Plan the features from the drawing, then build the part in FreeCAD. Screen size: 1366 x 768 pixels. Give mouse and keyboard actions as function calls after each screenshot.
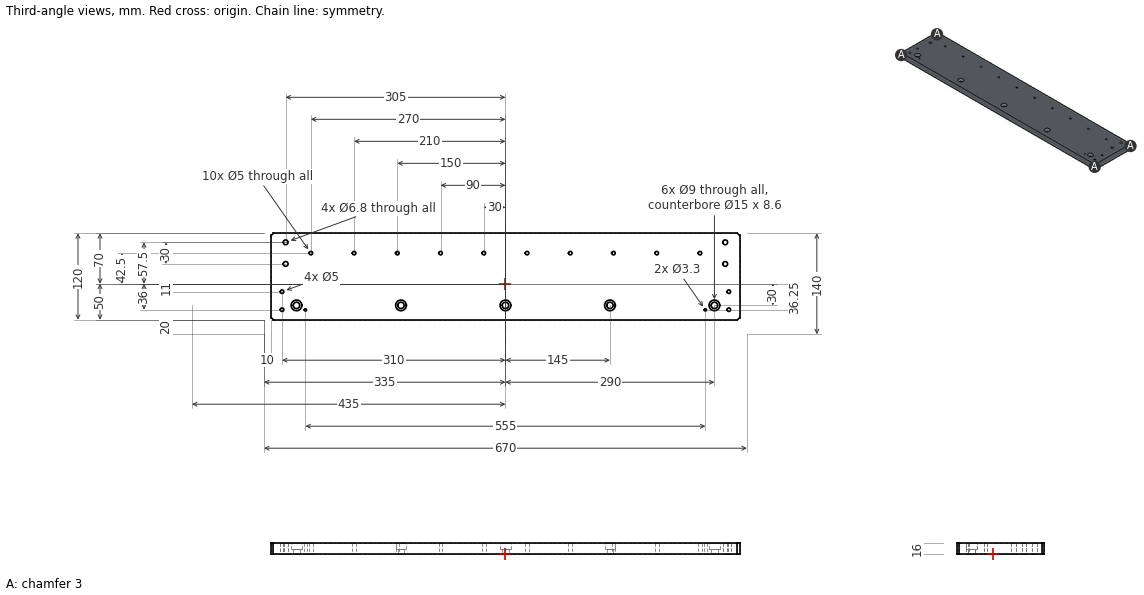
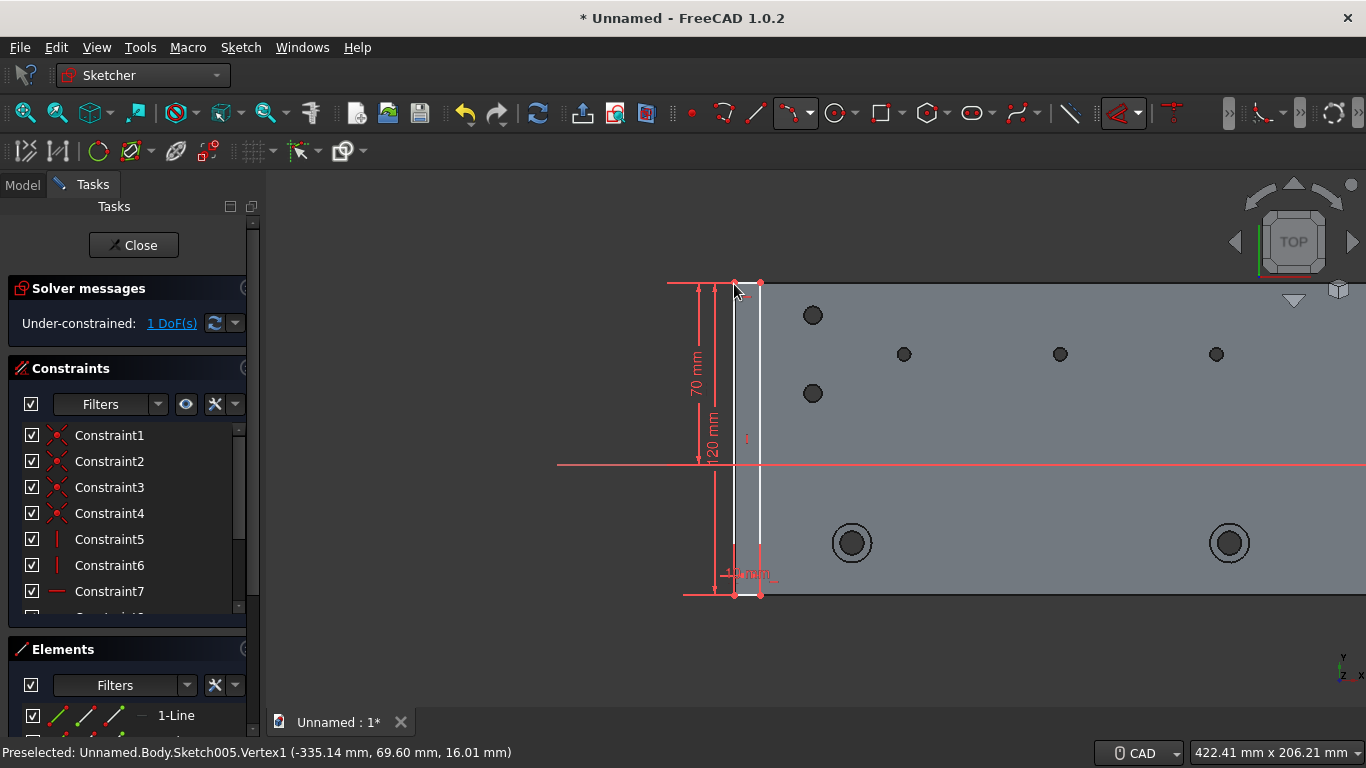
click(734, 283)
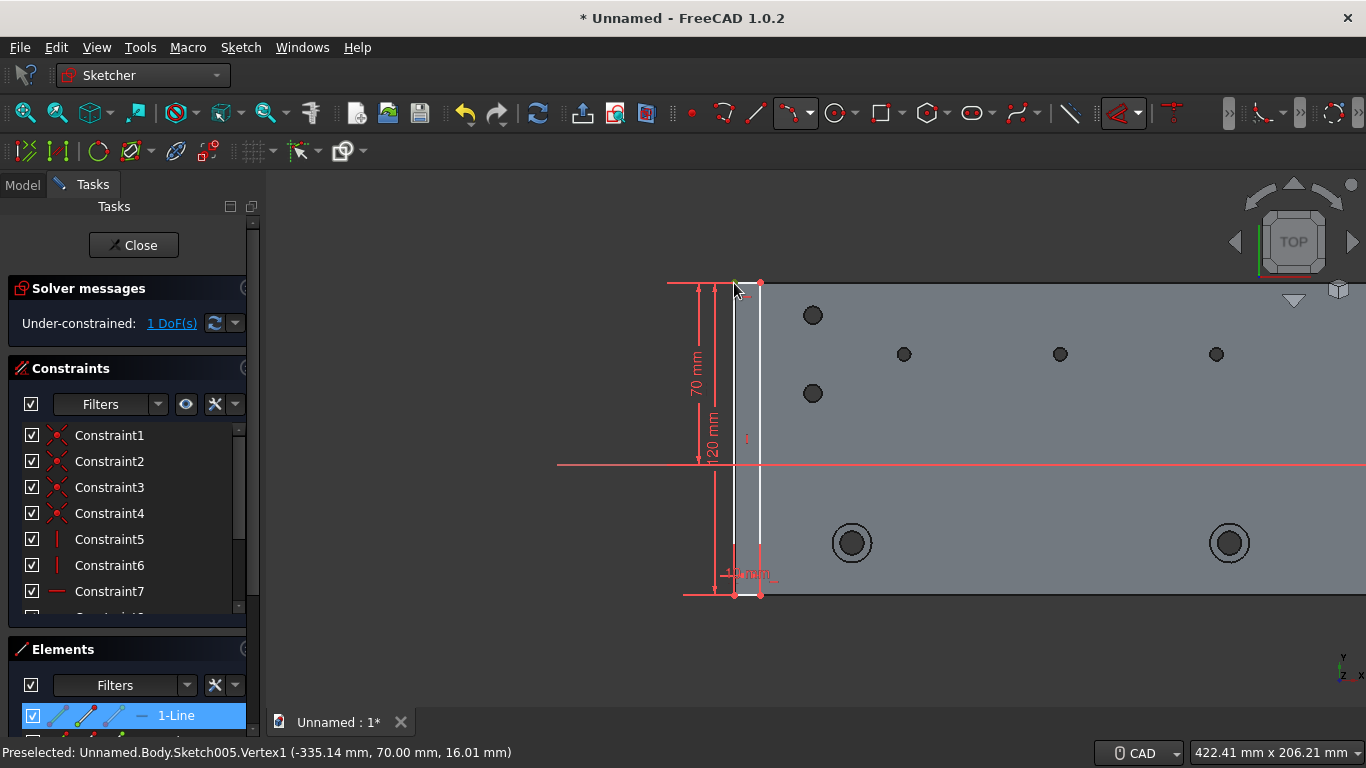
click(1140, 114)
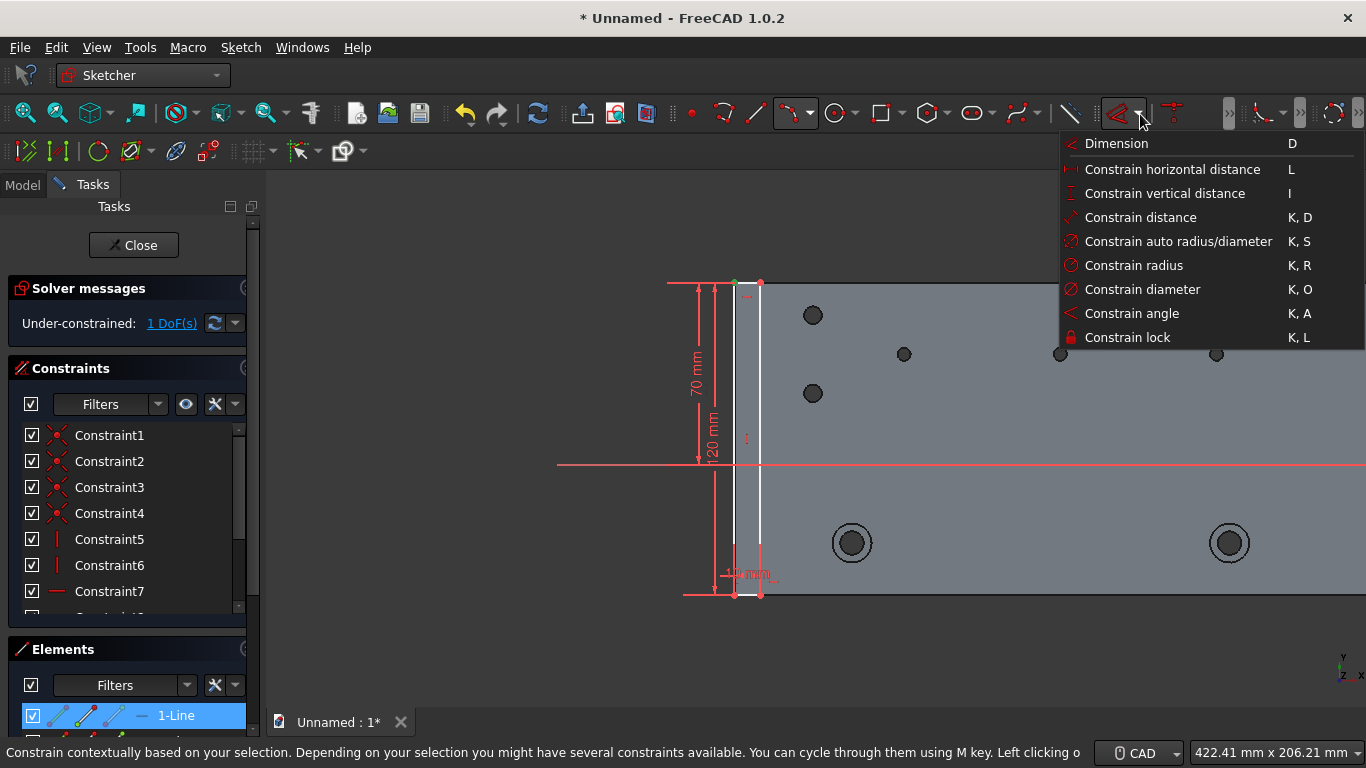
click(1212, 169)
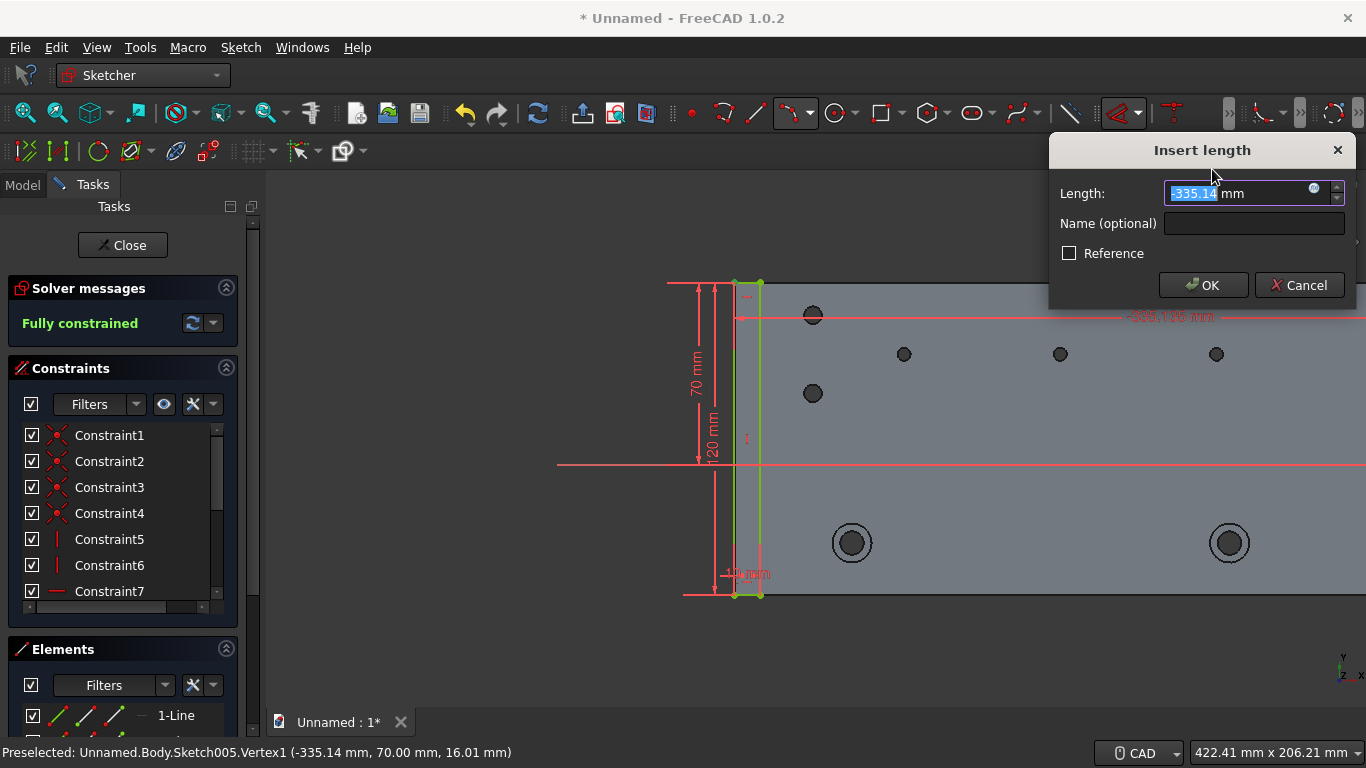
text(-335)
key(Return)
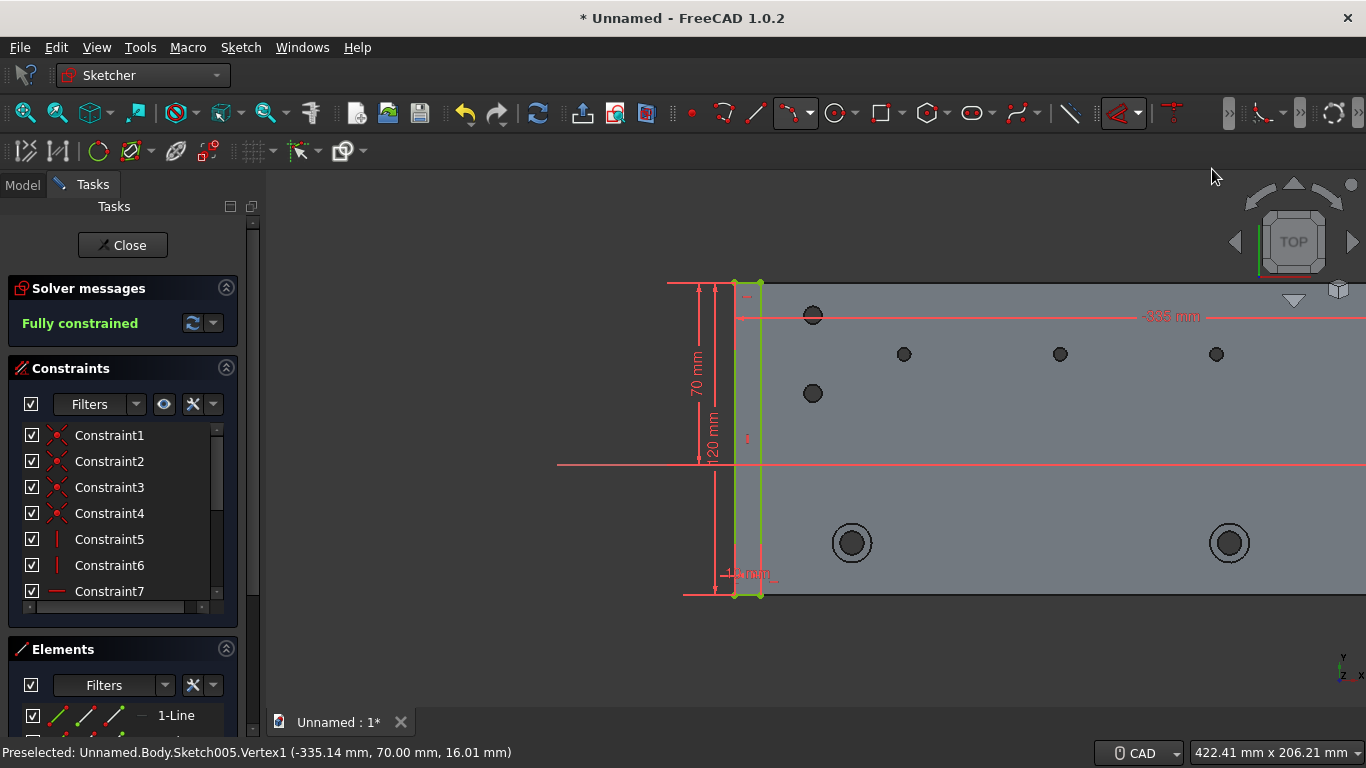
click(123, 245)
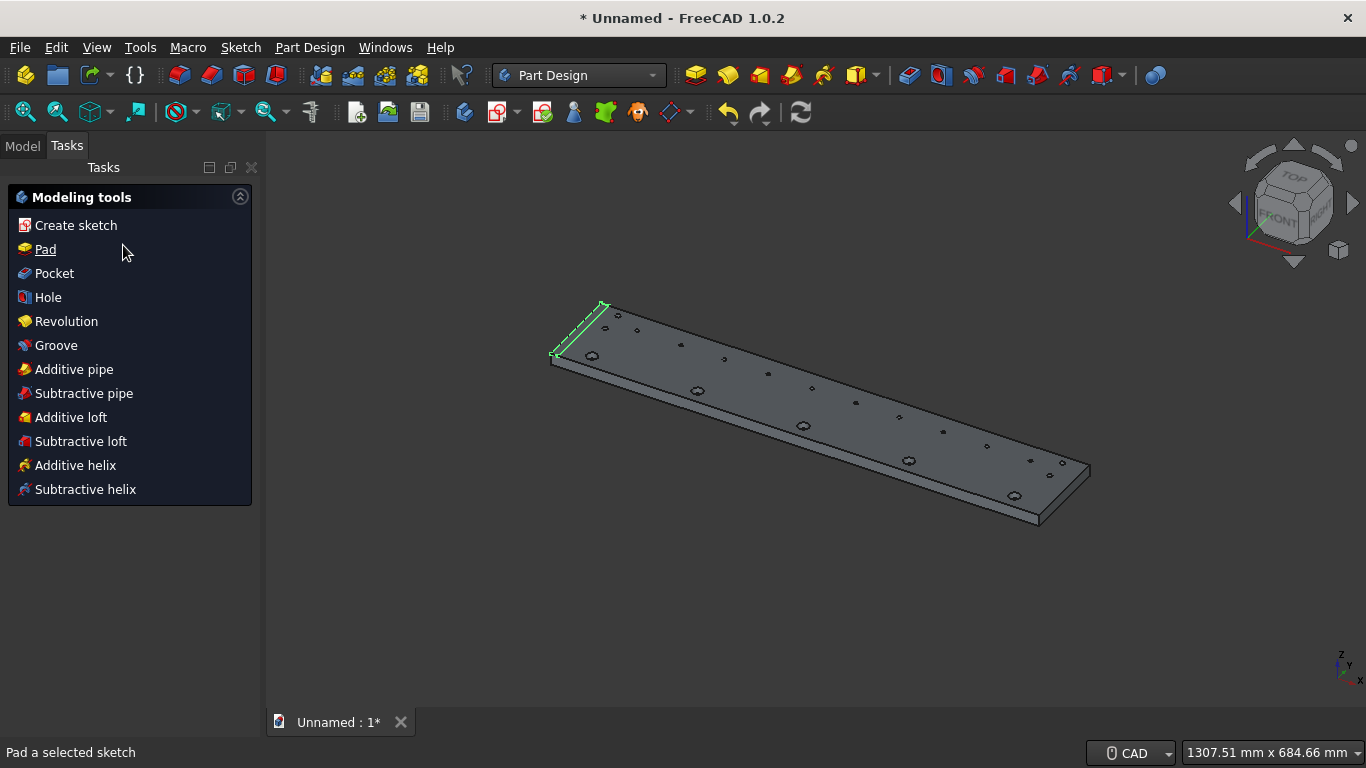
click(910, 76)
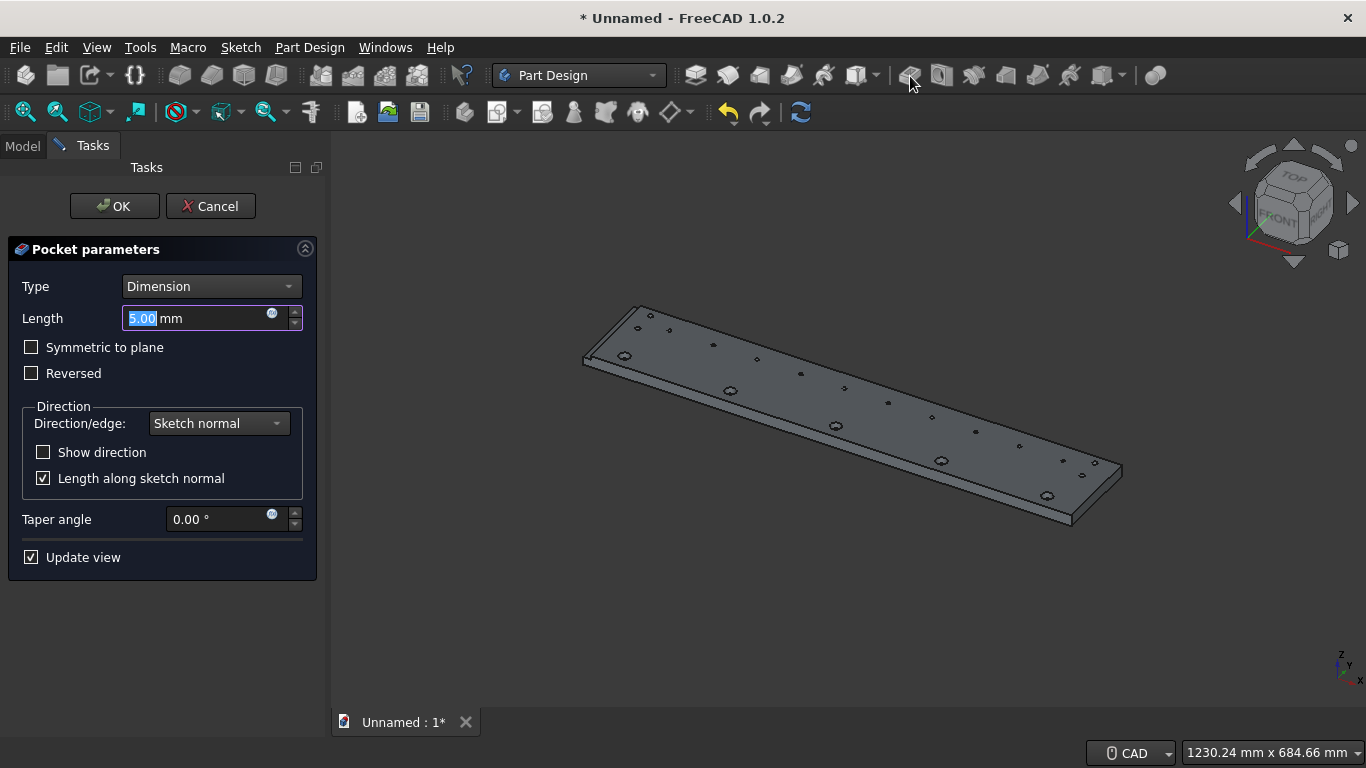
click(212, 286)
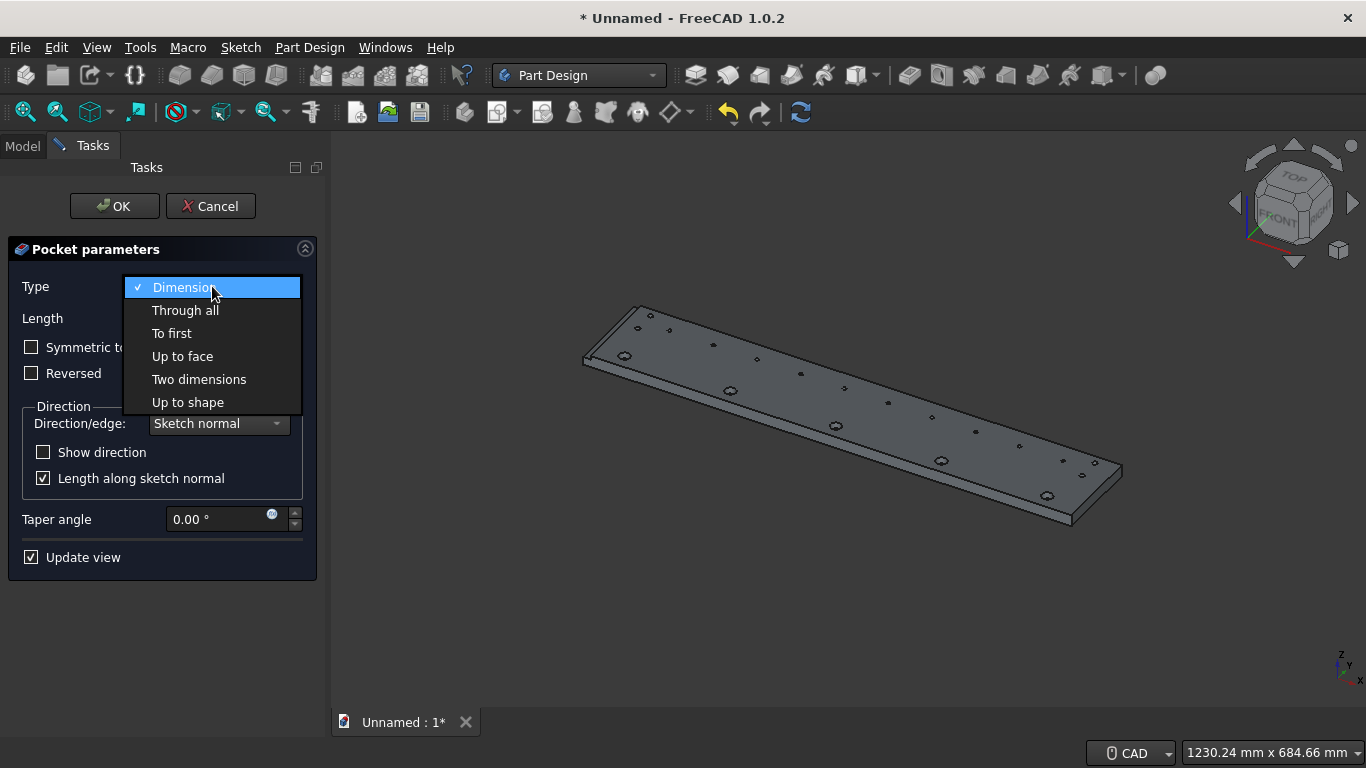
click(212, 310)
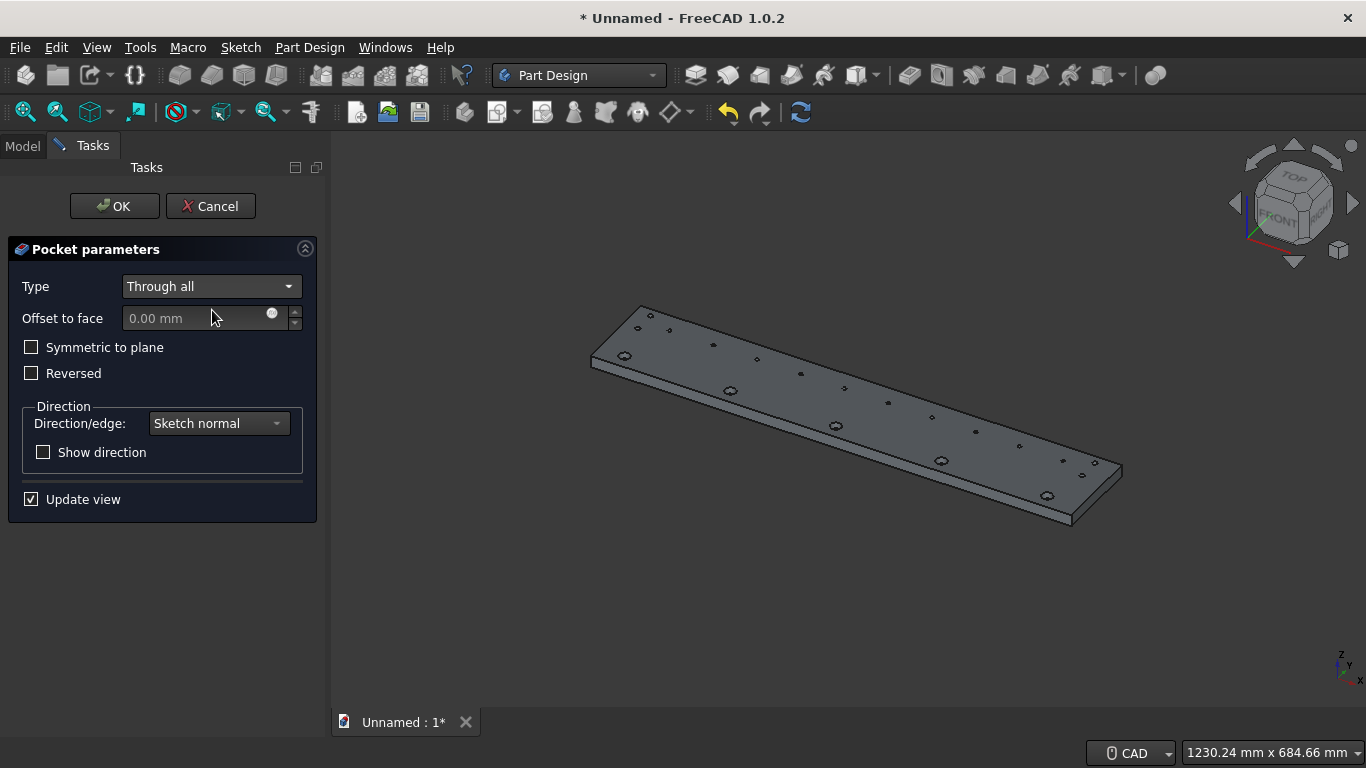
click(115, 206)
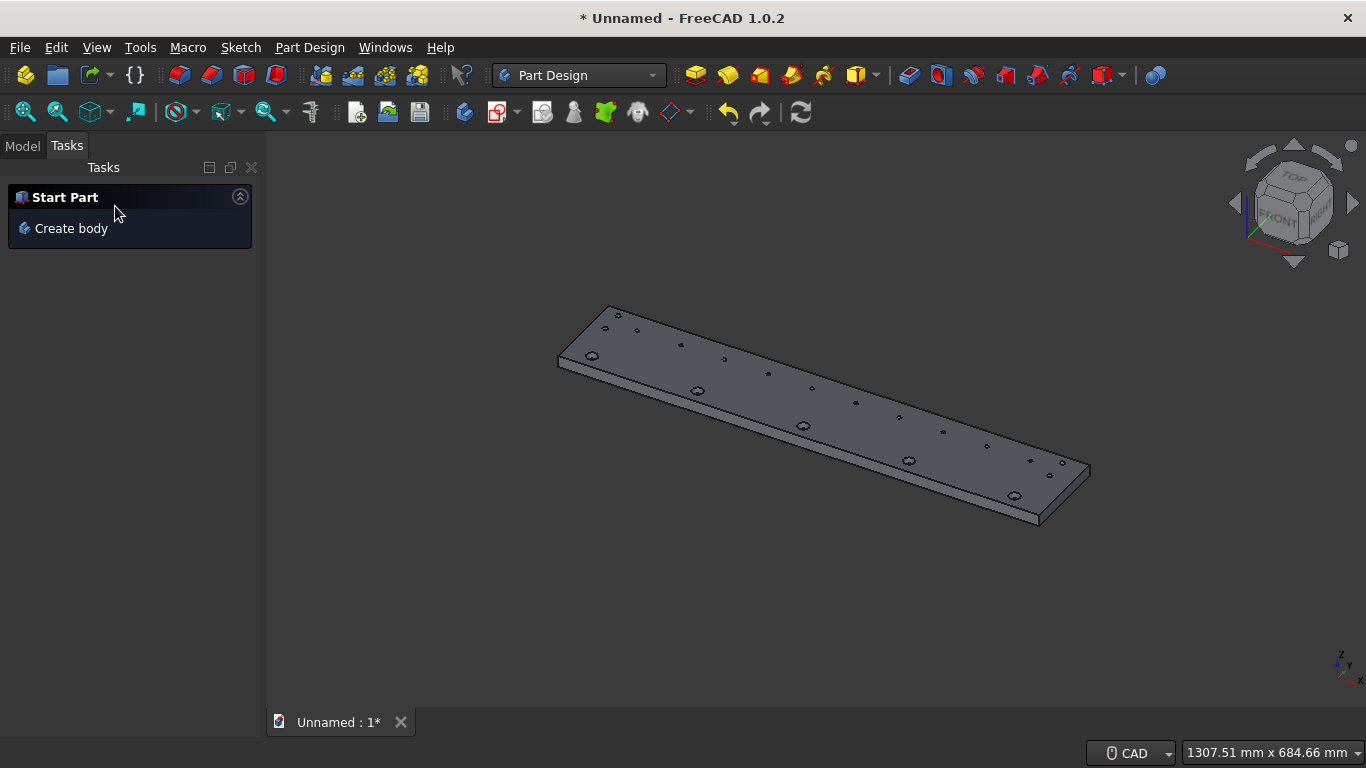
click(23, 145)